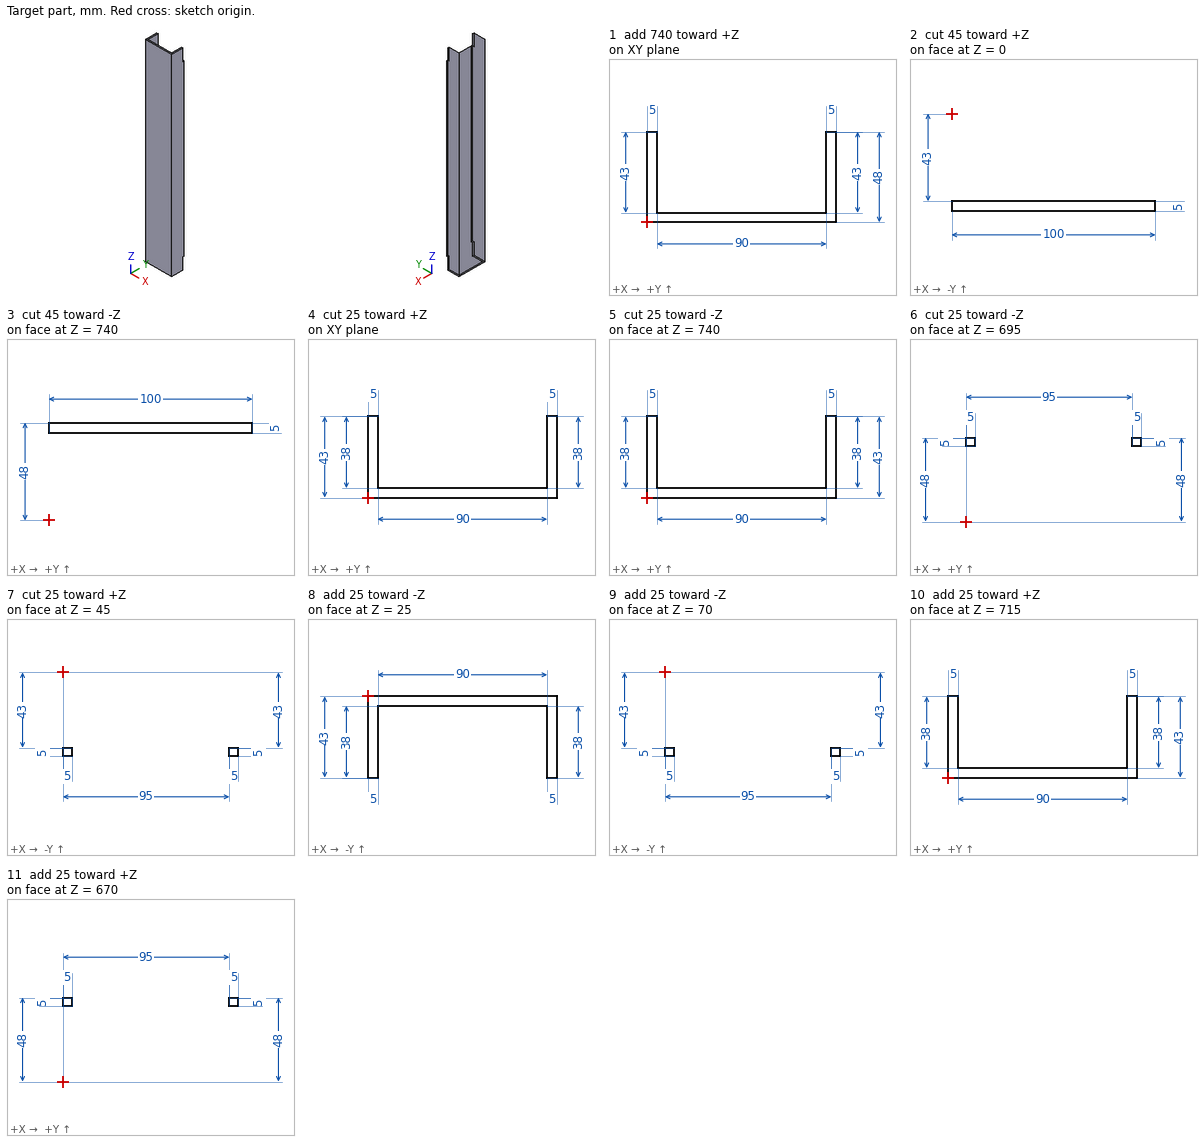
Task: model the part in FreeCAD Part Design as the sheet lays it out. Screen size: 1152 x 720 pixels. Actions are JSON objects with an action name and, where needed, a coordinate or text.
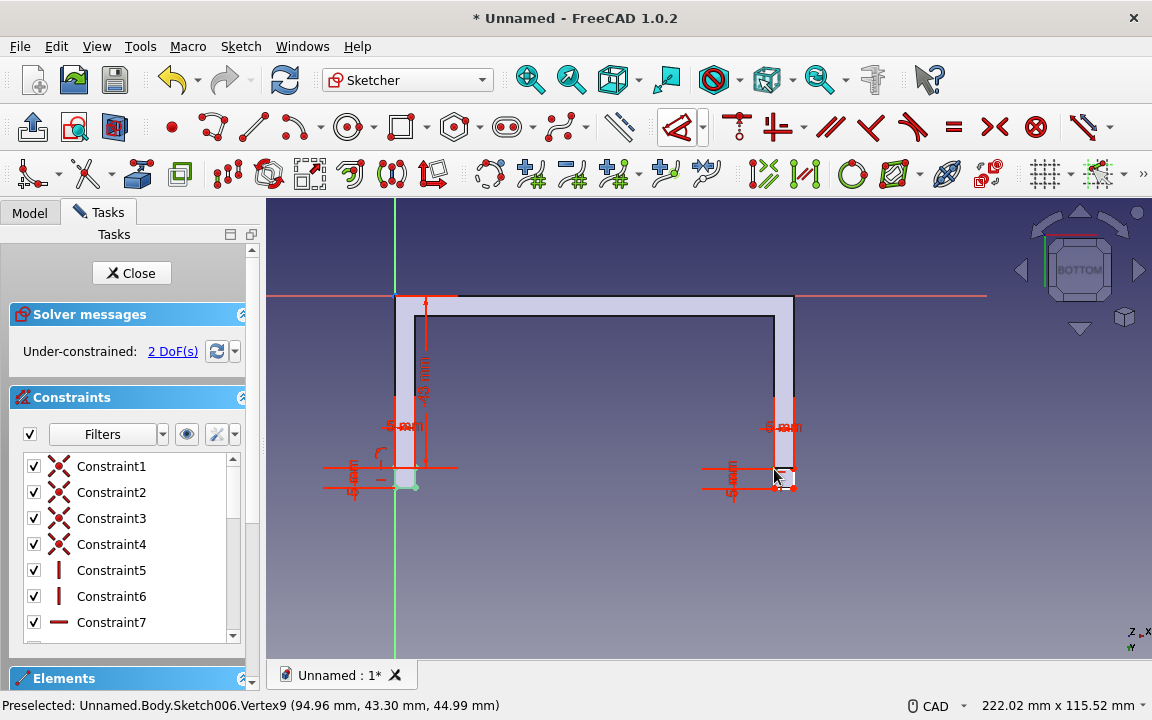
{"action": "key", "text": "l"}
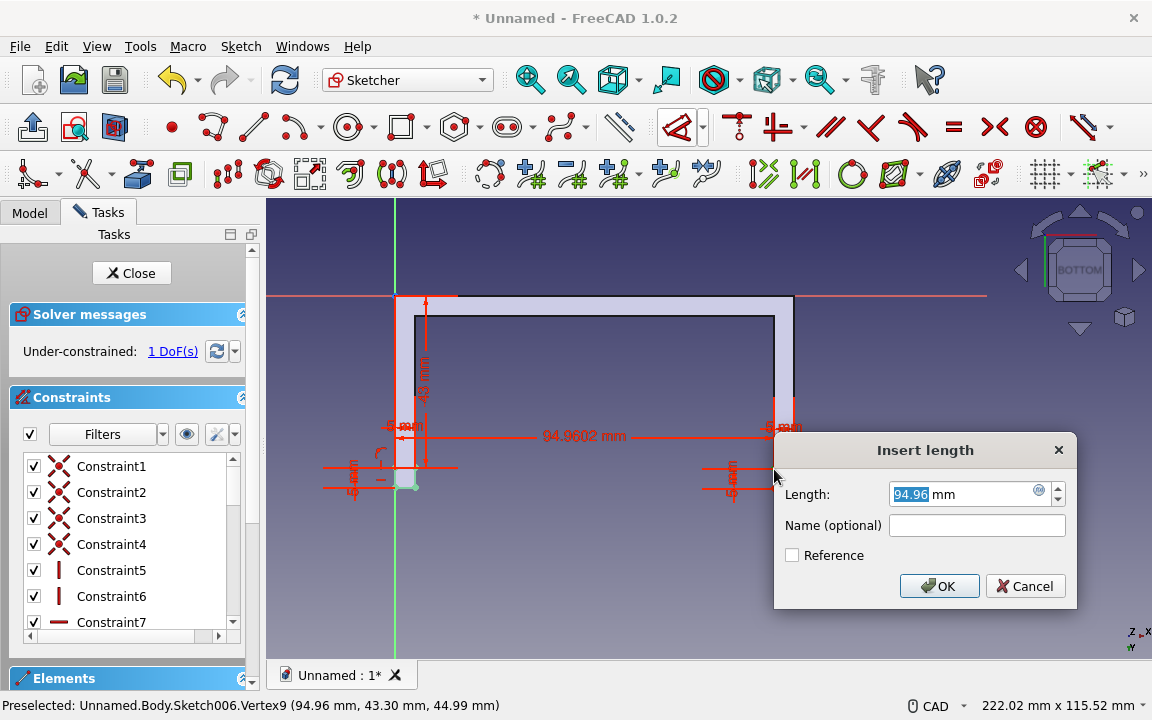
{"action": "type", "text": "95"}
{"action": "key", "text": "Return"}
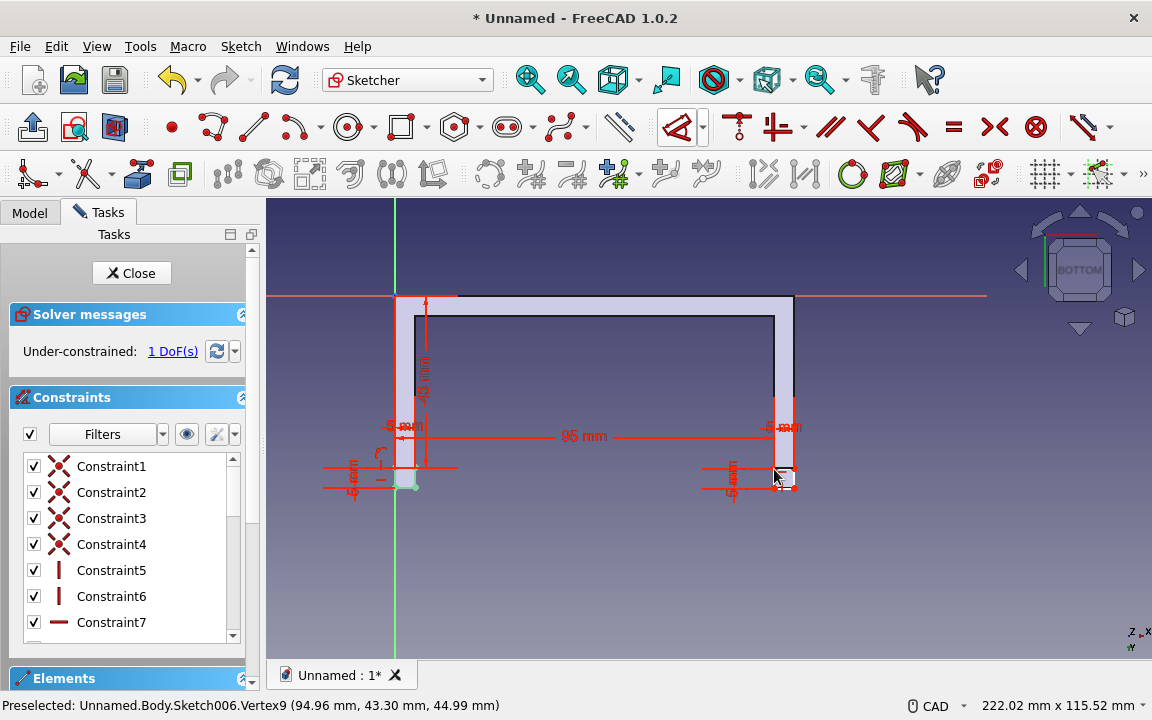
{"action": "left_click", "coordinate": [774, 469]}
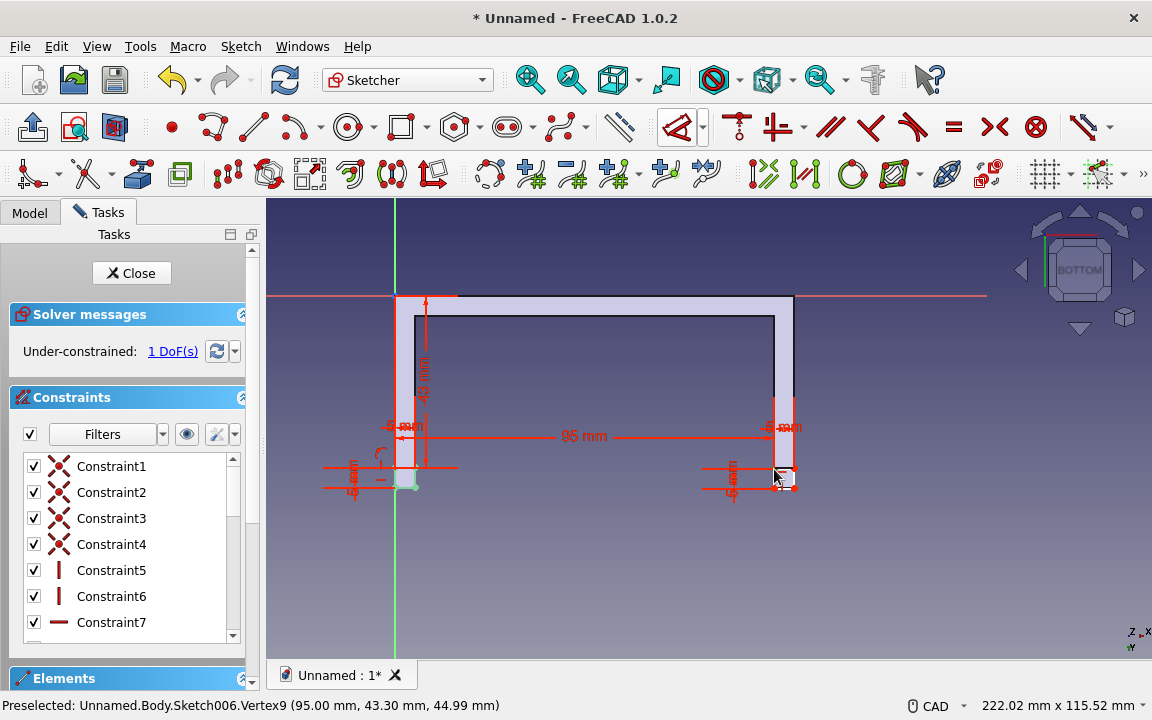
{"action": "key", "text": "i"}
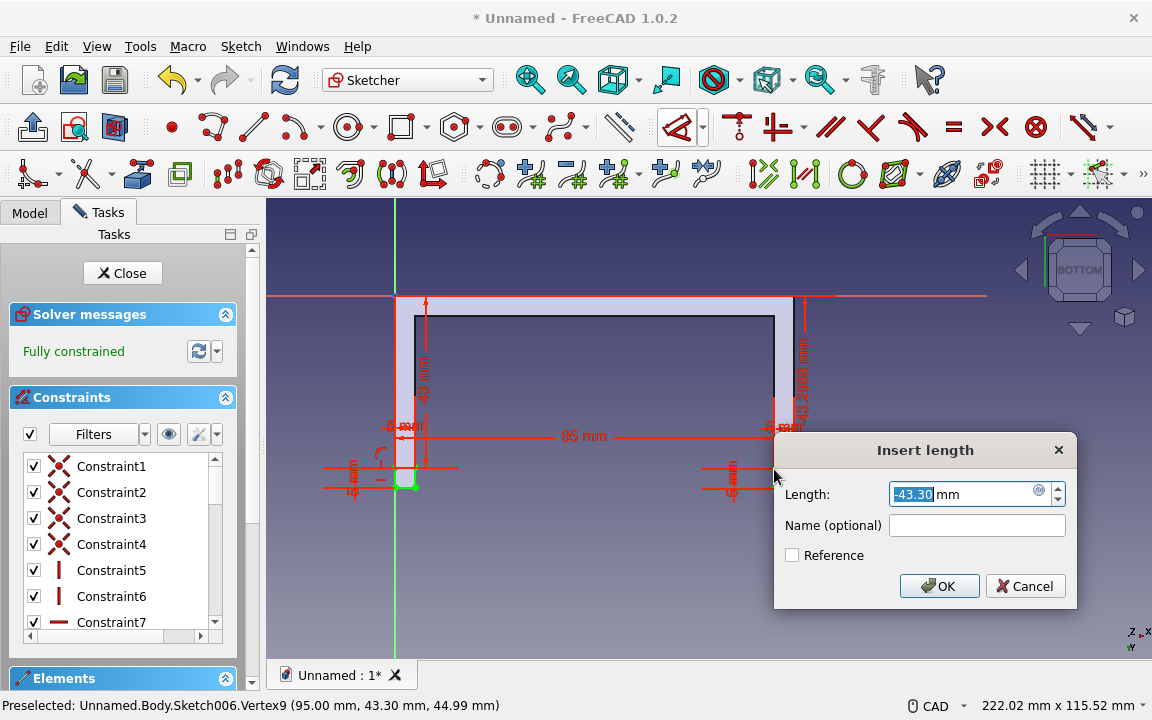
{"action": "type", "text": "-43"}
{"action": "key", "text": "Return"}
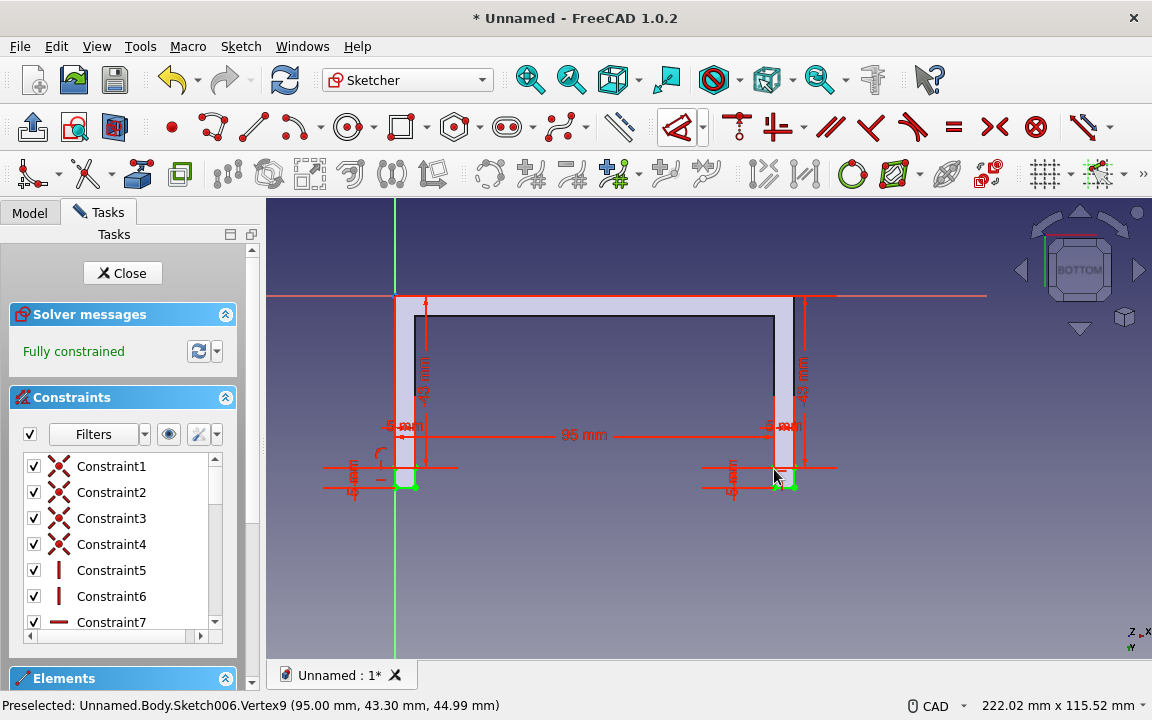
{"action": "left_click", "coordinate": [123, 273]}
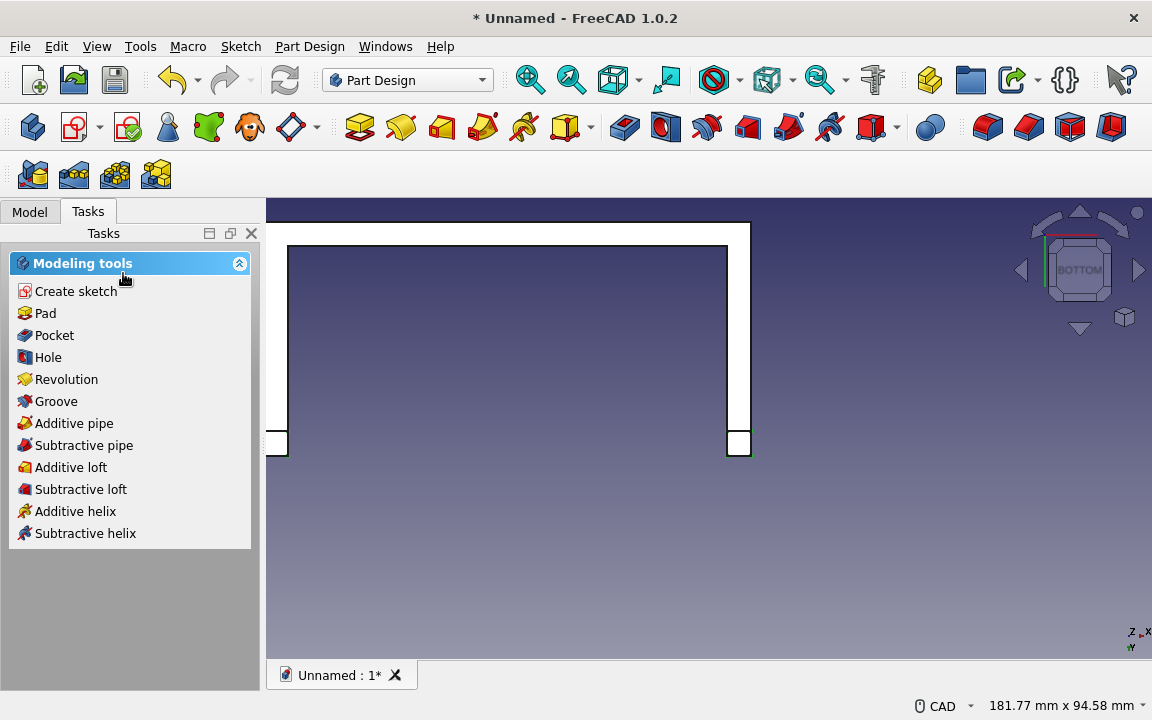
{"action": "left_click", "coordinate": [625, 128]}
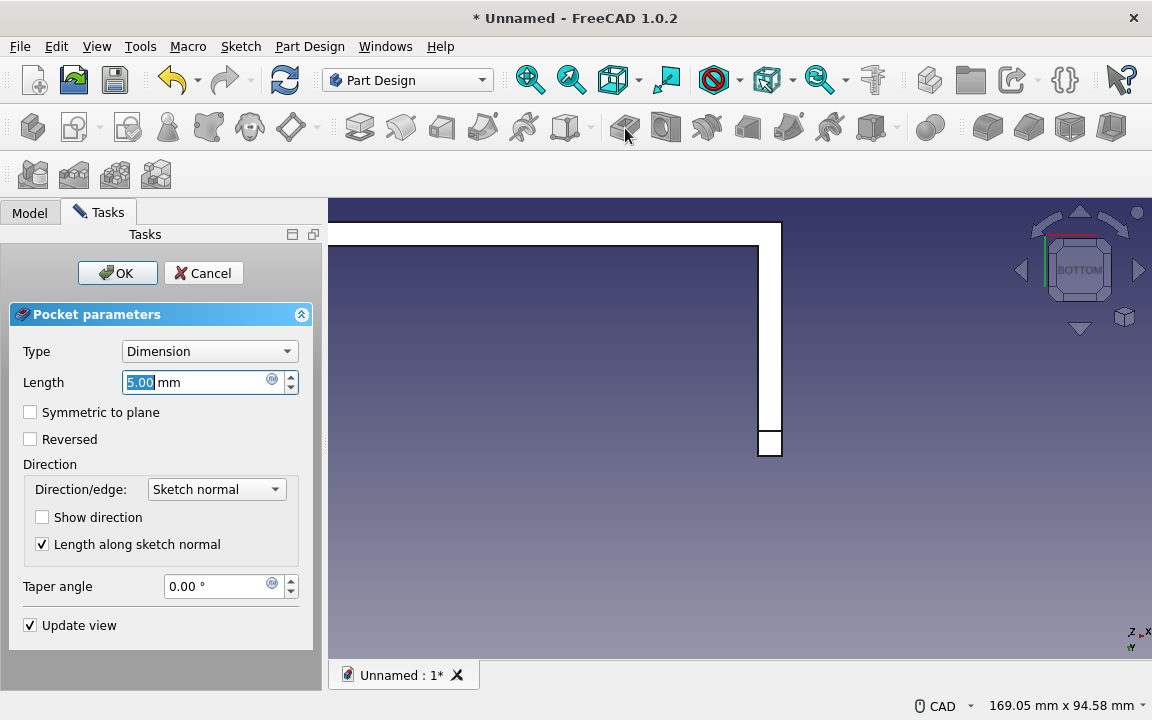
{"action": "type", "text": "25"}
{"action": "key", "text": "Tab"}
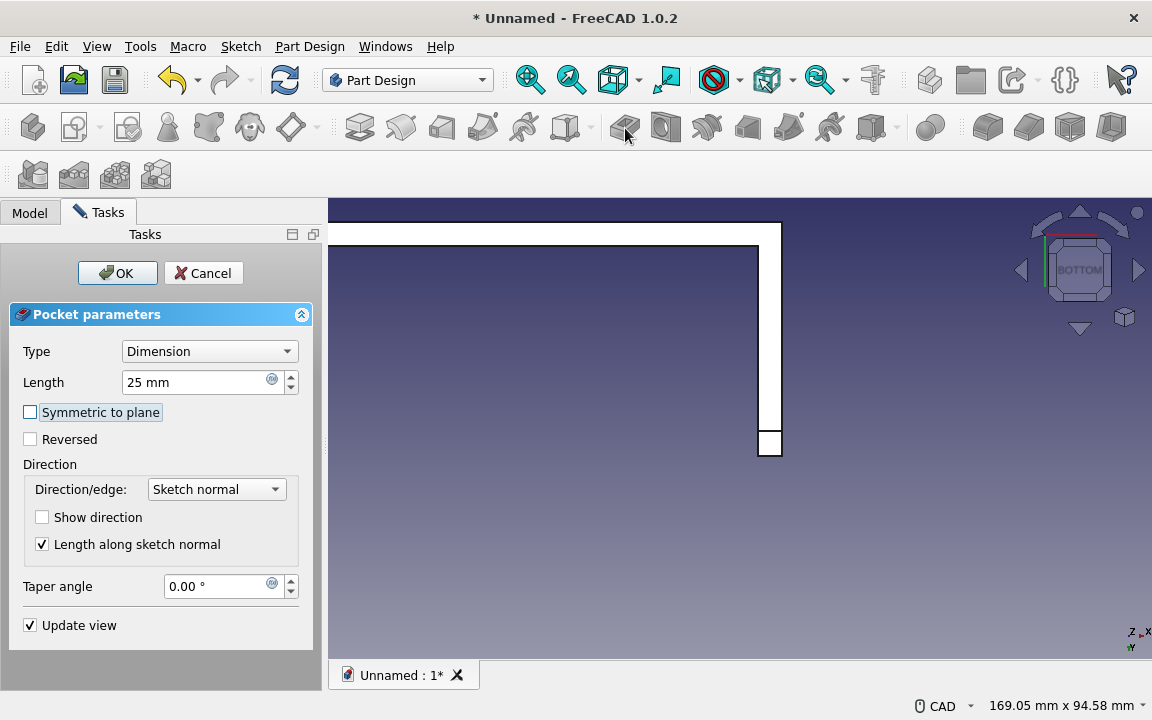
{"action": "left_click", "coordinate": [118, 273]}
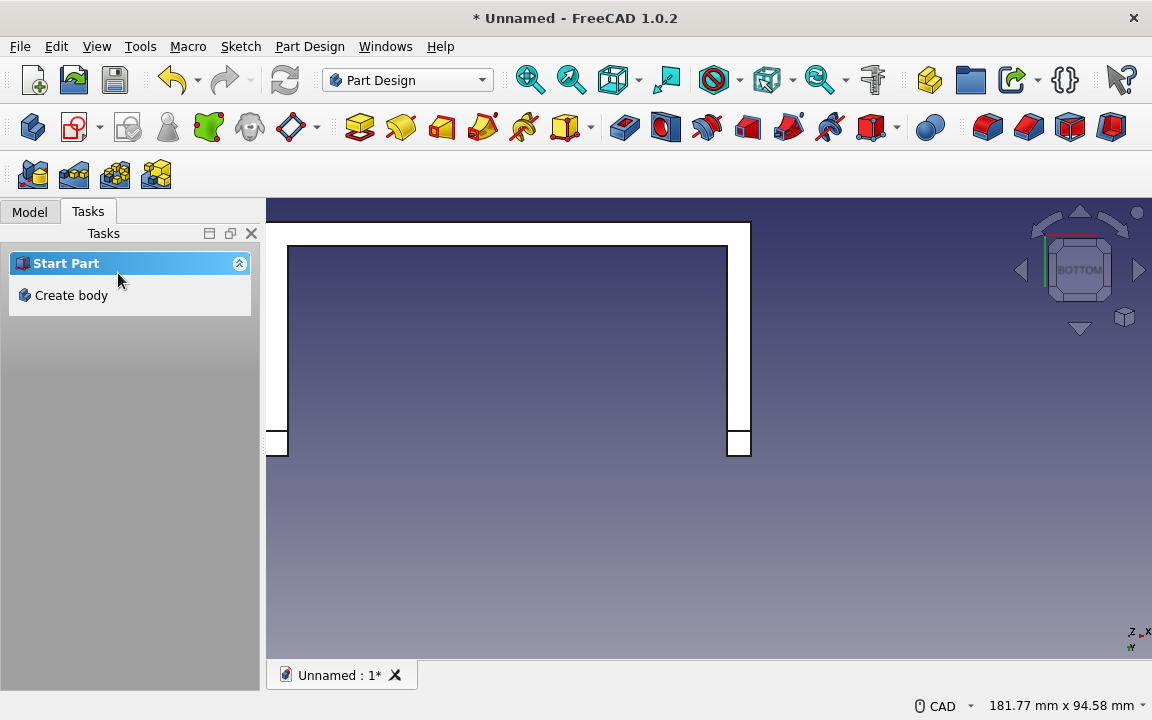
{"action": "left_click", "coordinate": [531, 80]}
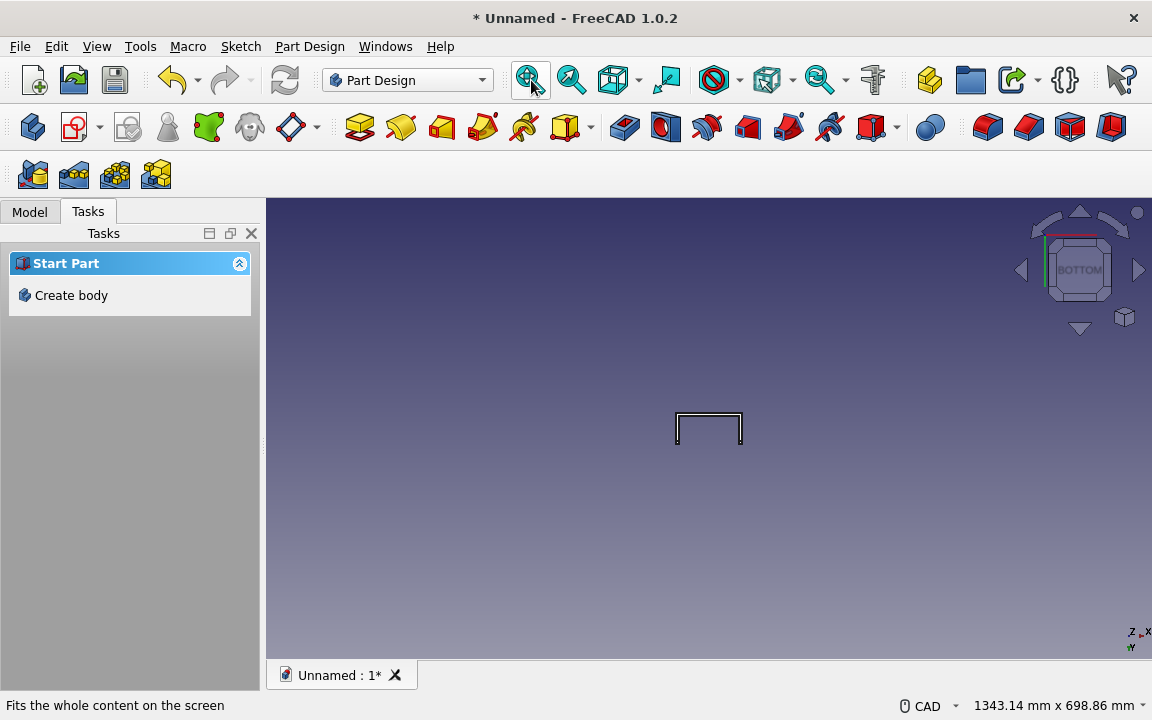
{"action": "scroll", "coordinate": [737, 414], "scroll_direction": "up", "scroll_amount": 12}